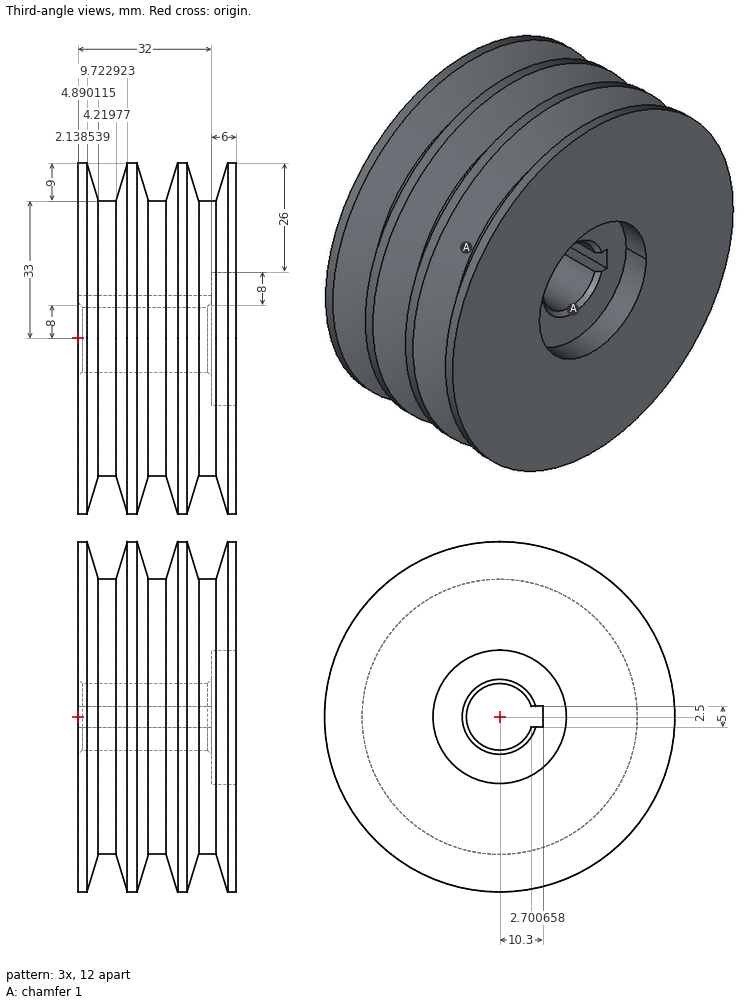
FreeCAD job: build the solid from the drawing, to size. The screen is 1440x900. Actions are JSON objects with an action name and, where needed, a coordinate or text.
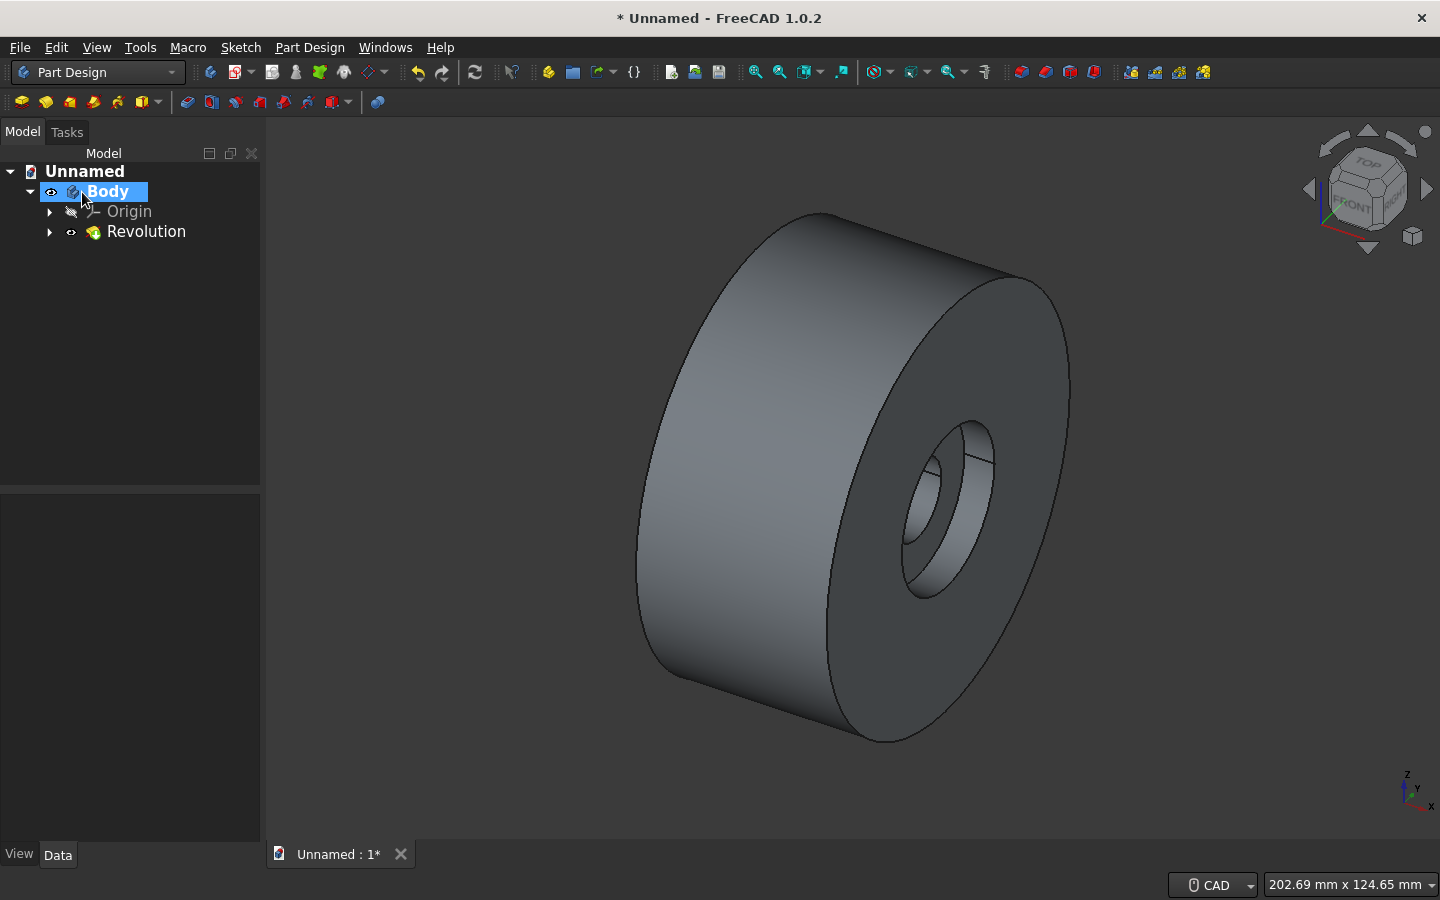
{"action": "left_click", "coordinate": [236, 72]}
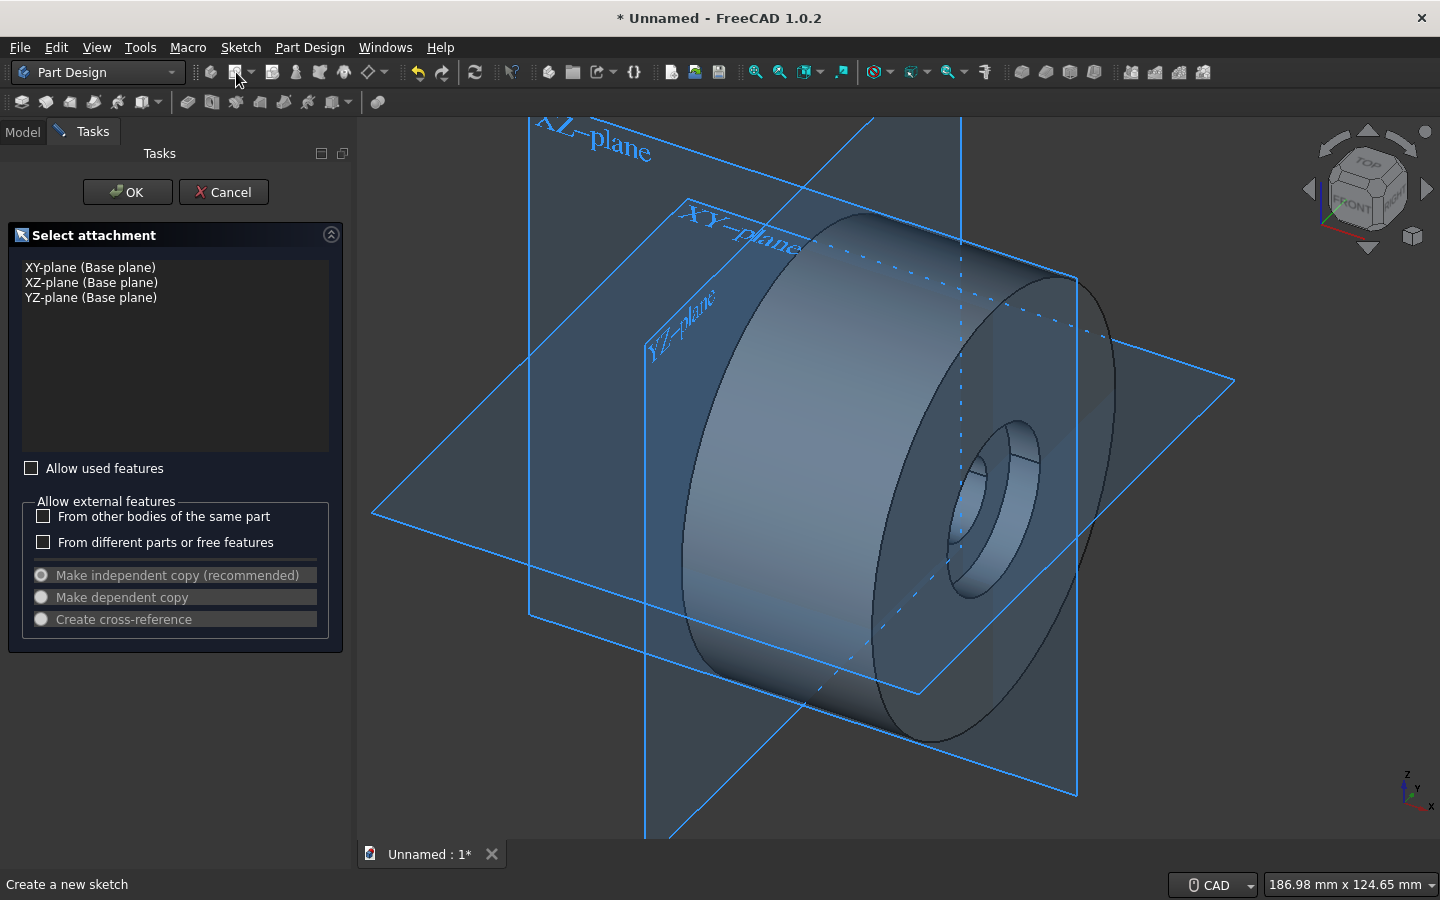
{"action": "left_click", "coordinate": [82, 268]}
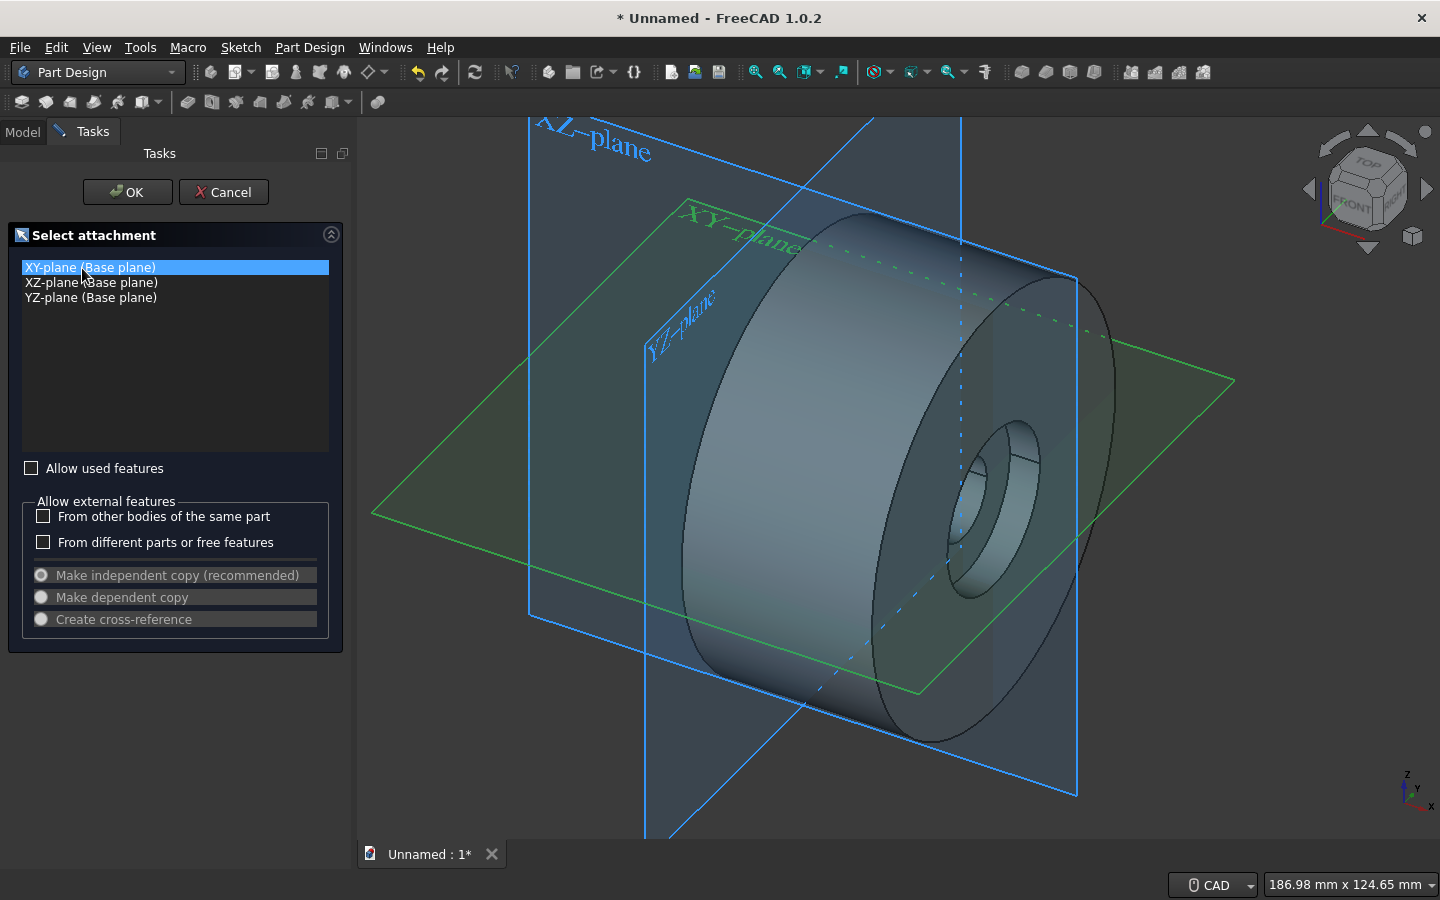
{"action": "left_click", "coordinate": [128, 192]}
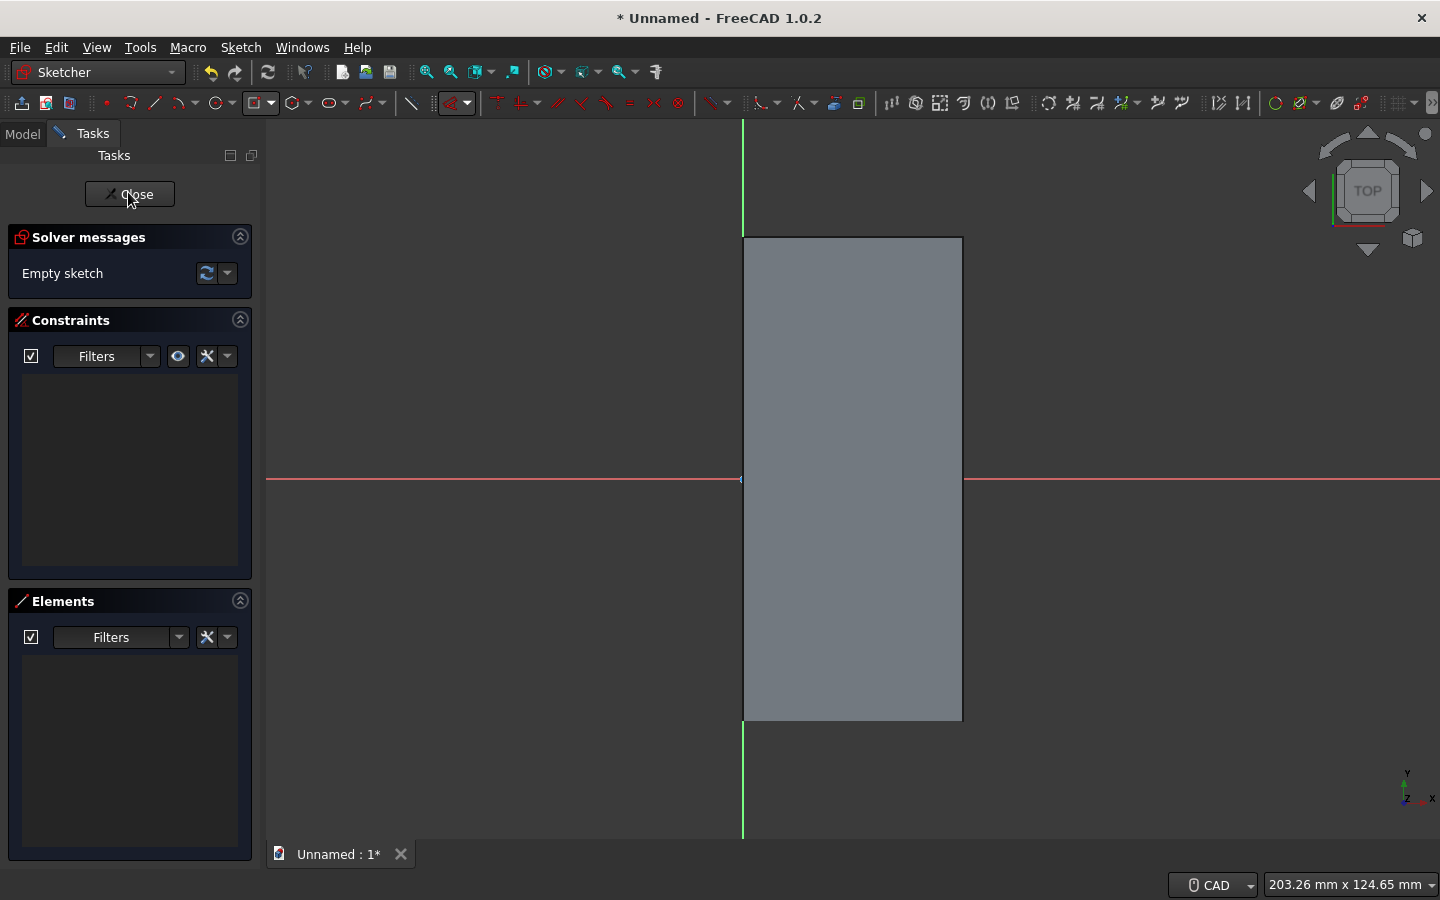
{"action": "left_click", "coordinate": [70, 104]}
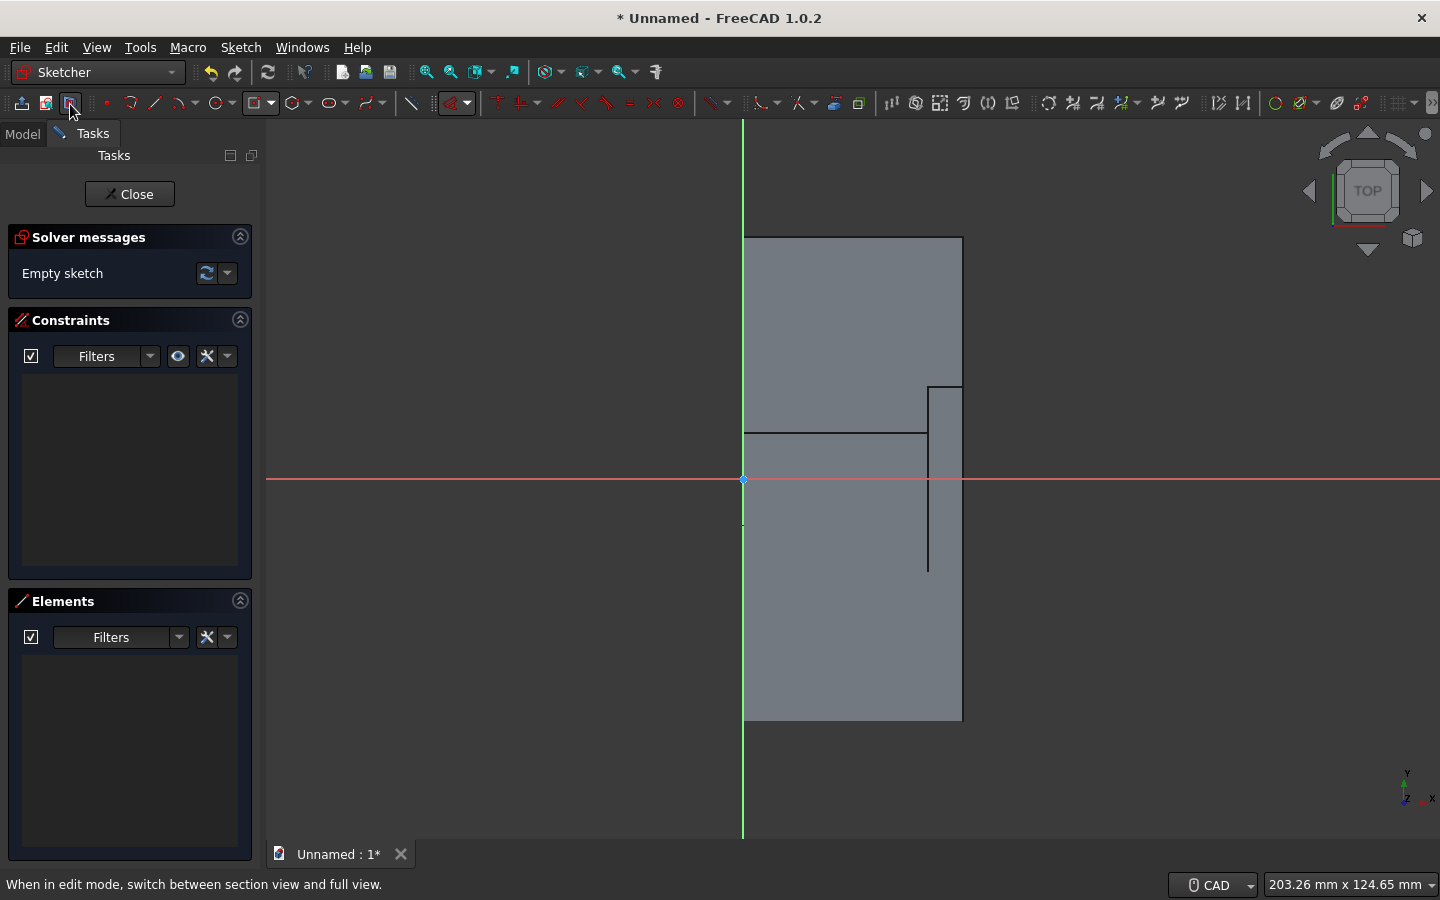
{"action": "scroll", "coordinate": [784, 236], "scroll_direction": "up", "scroll_amount": 11}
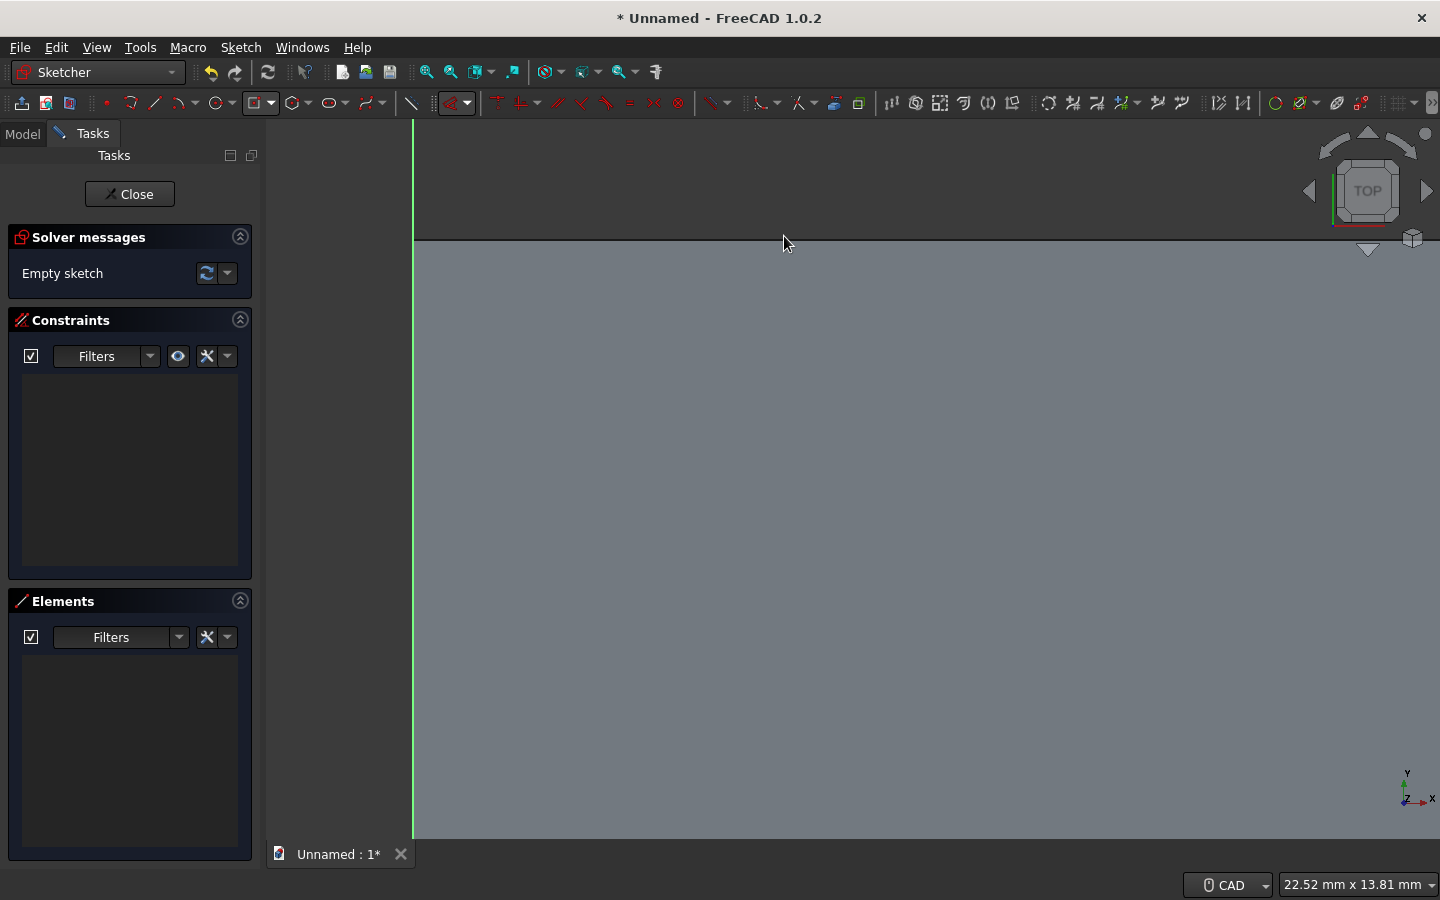
{"action": "key", "text": "g m"}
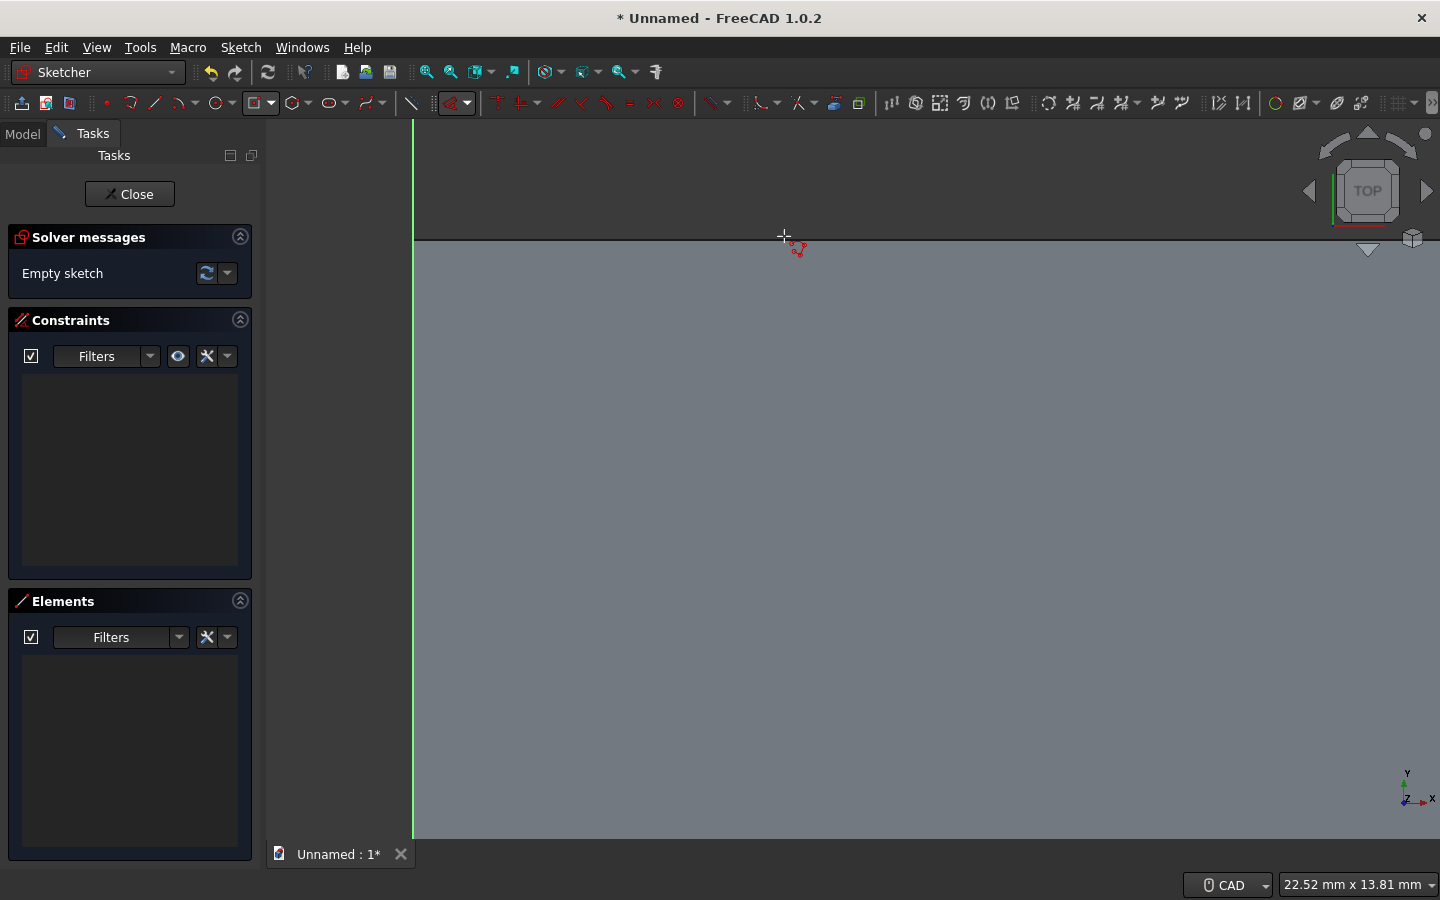
{"action": "left_click", "coordinate": [668, 709]}
{"action": "left_click", "coordinate": [888, 709]}
{"action": "left_click", "coordinate": [1031, 240]}
{"action": "left_click", "coordinate": [524, 240]}
{"action": "left_click", "coordinate": [668, 710]}
{"action": "key", "text": "Escape"}
{"action": "key", "text": "Escape"}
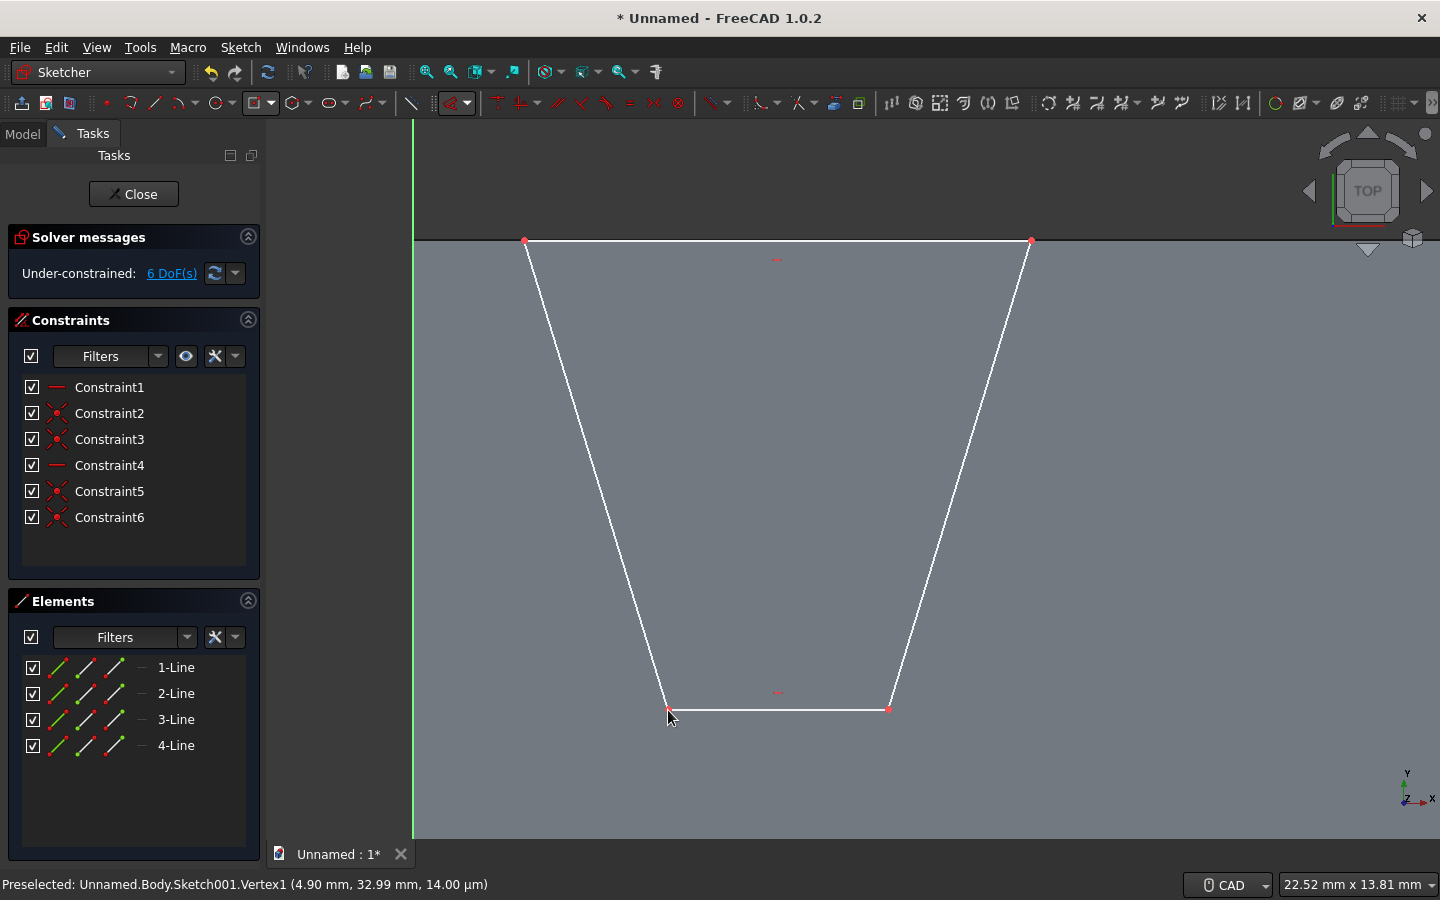
{"action": "key", "text": "d"}